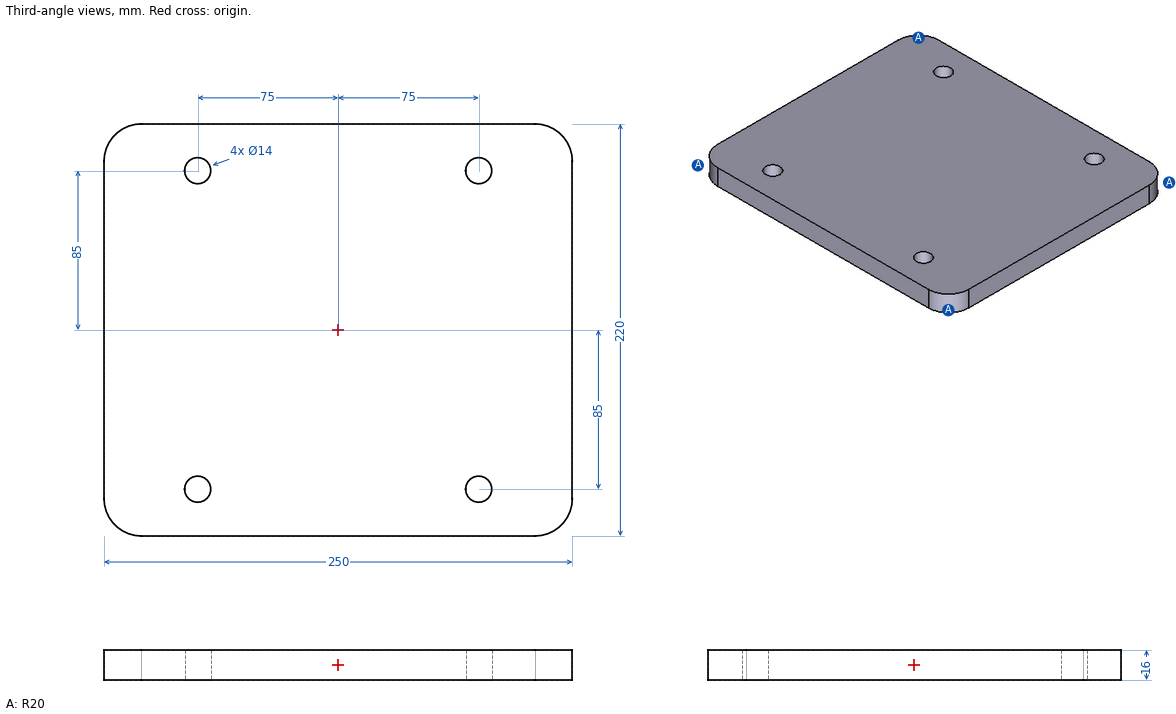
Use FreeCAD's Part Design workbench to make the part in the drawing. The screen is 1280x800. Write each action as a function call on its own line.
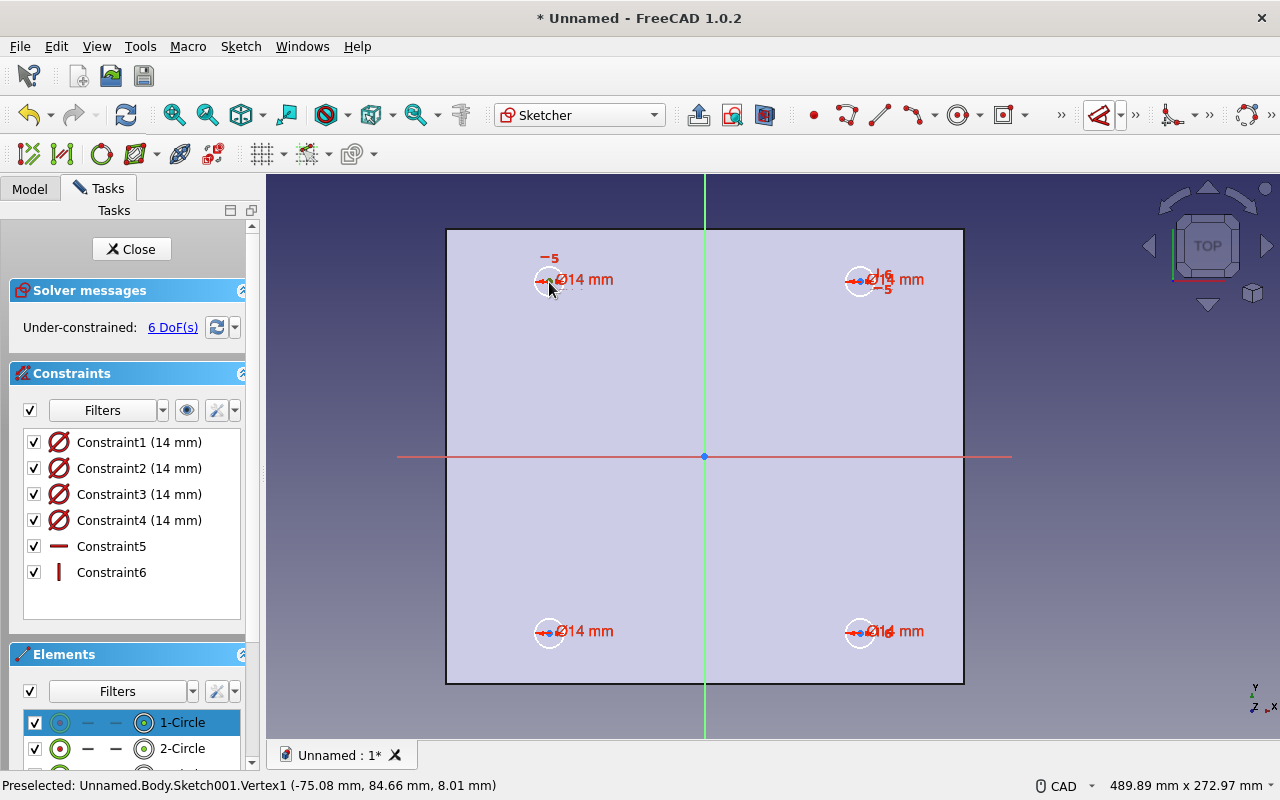
click(550, 633)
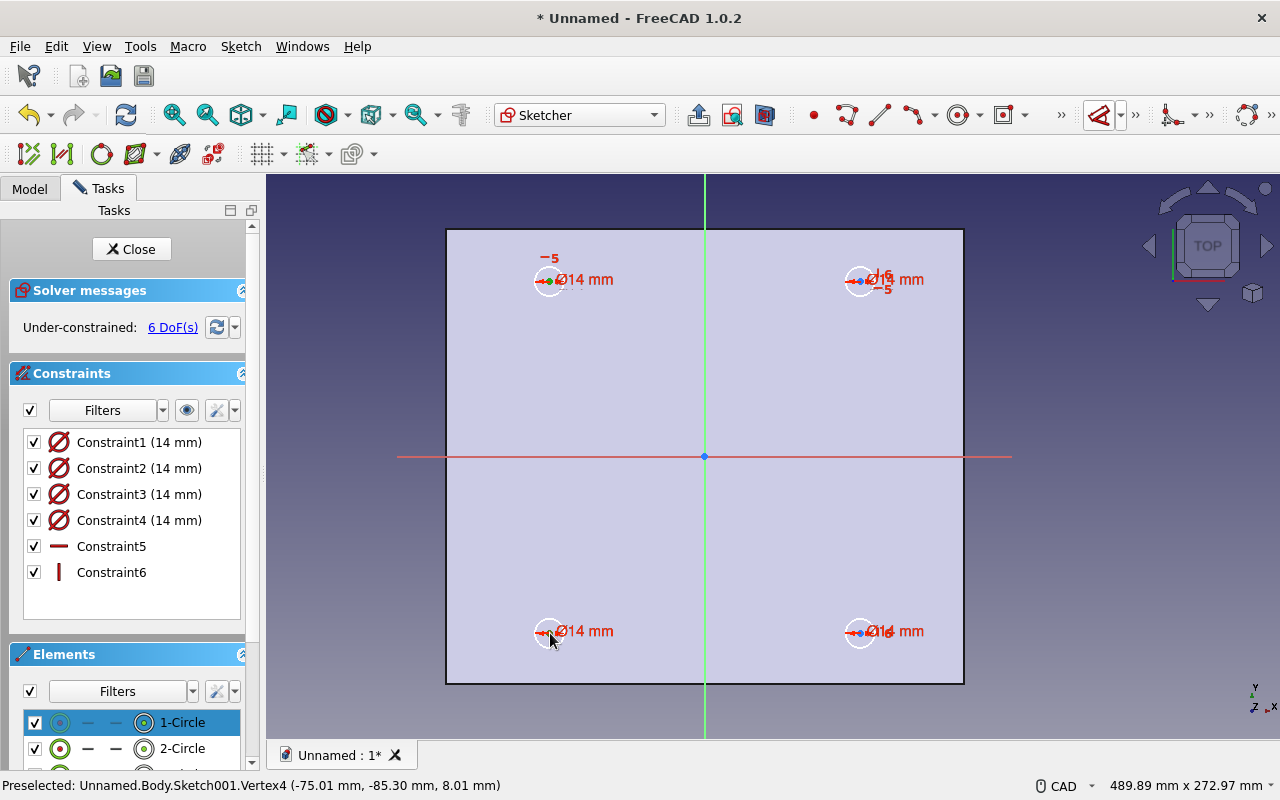
key(v)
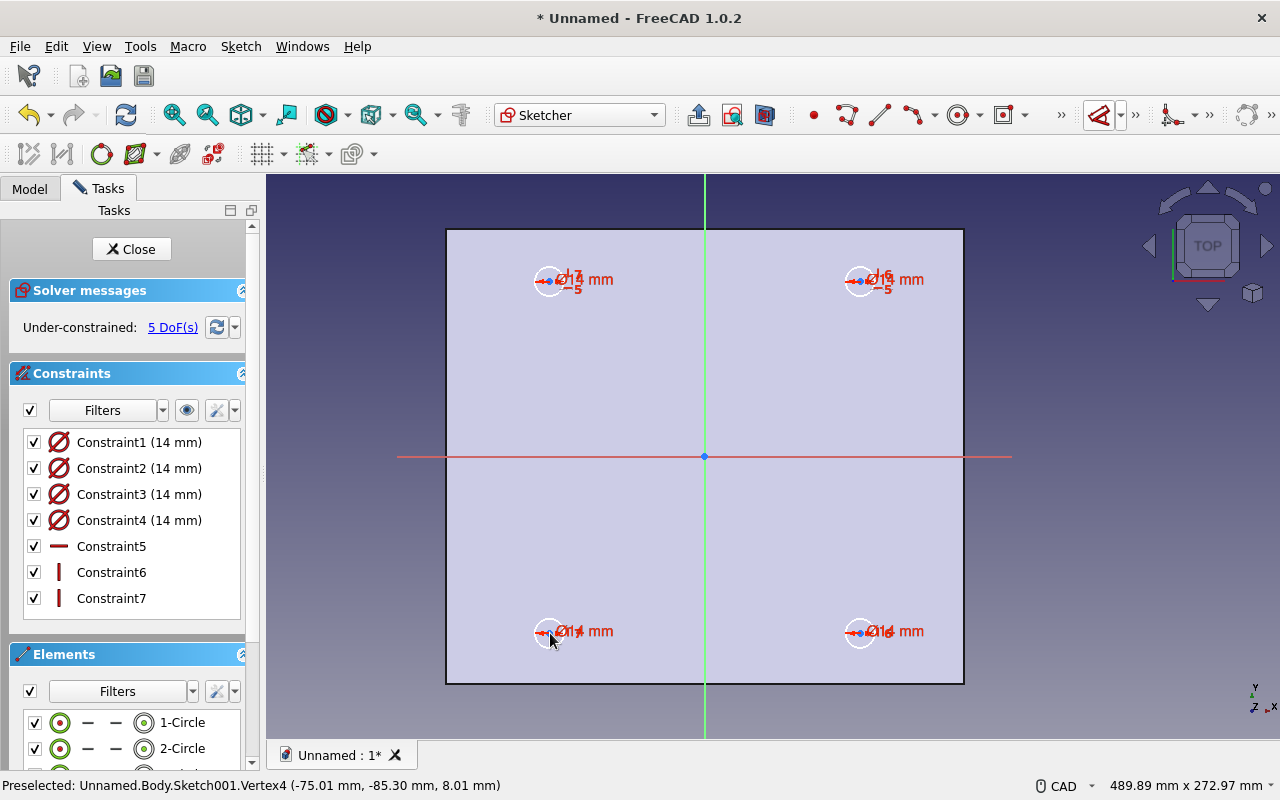
click(860, 633)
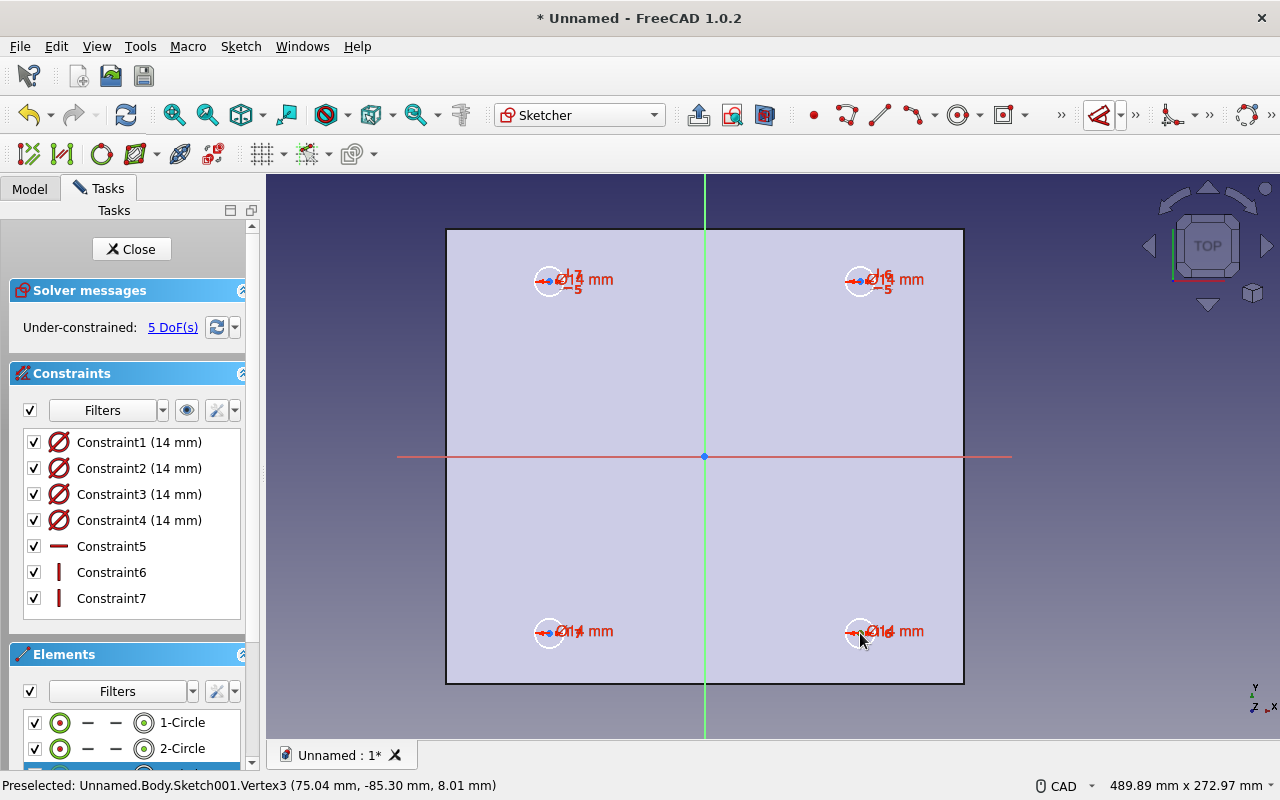
click(549, 633)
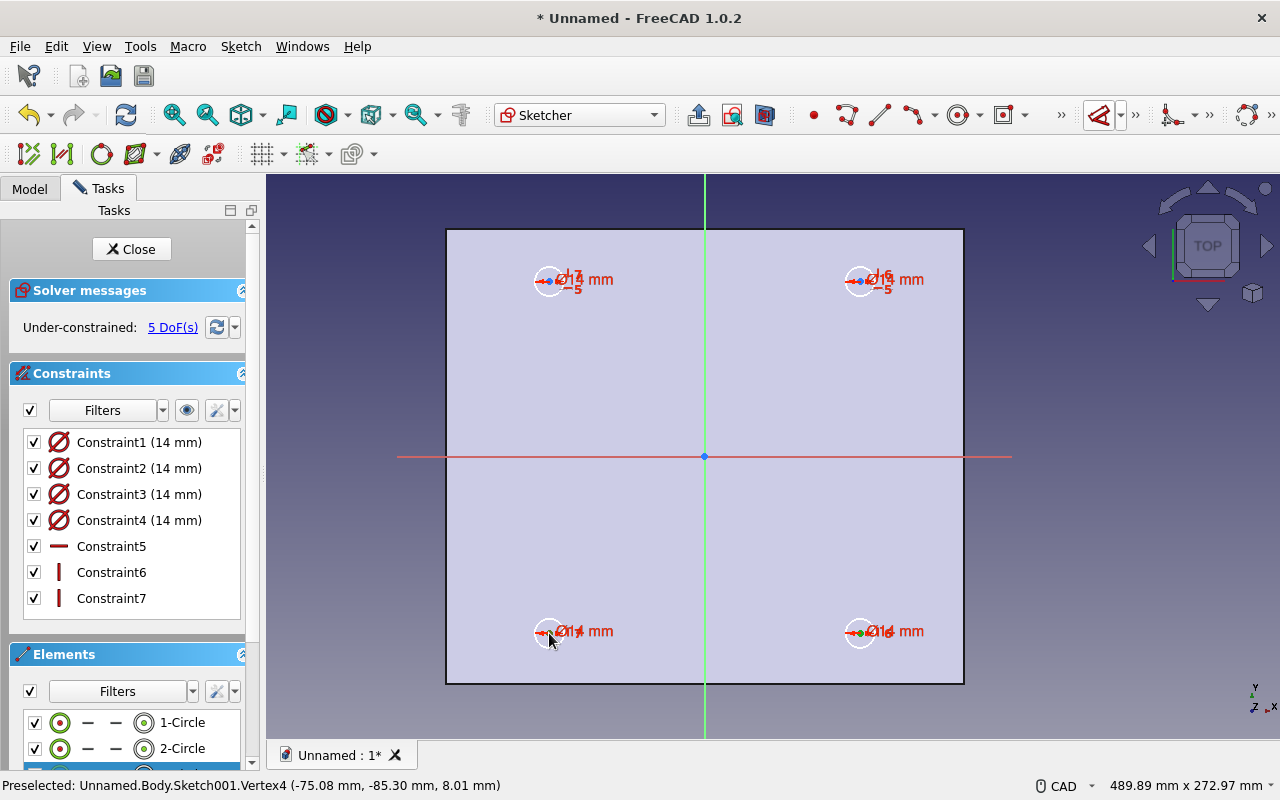
key(h)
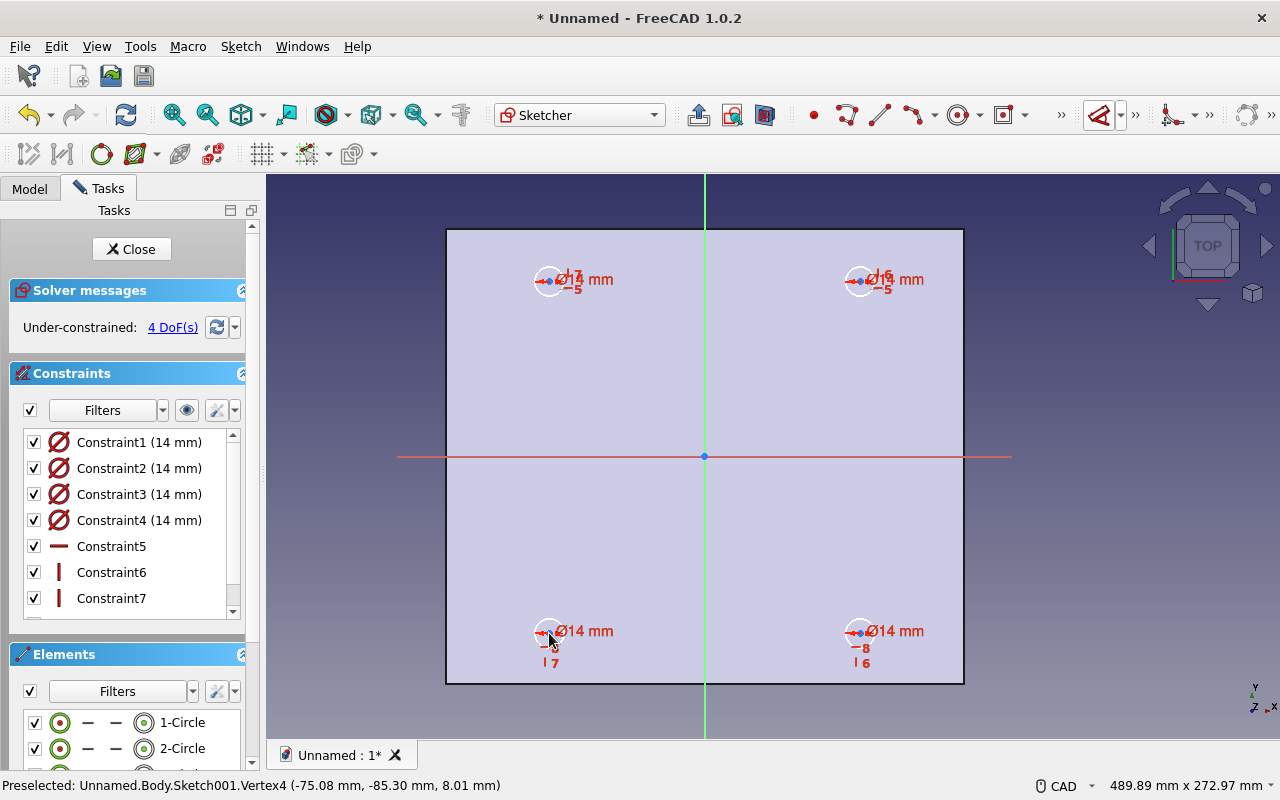
click(549, 282)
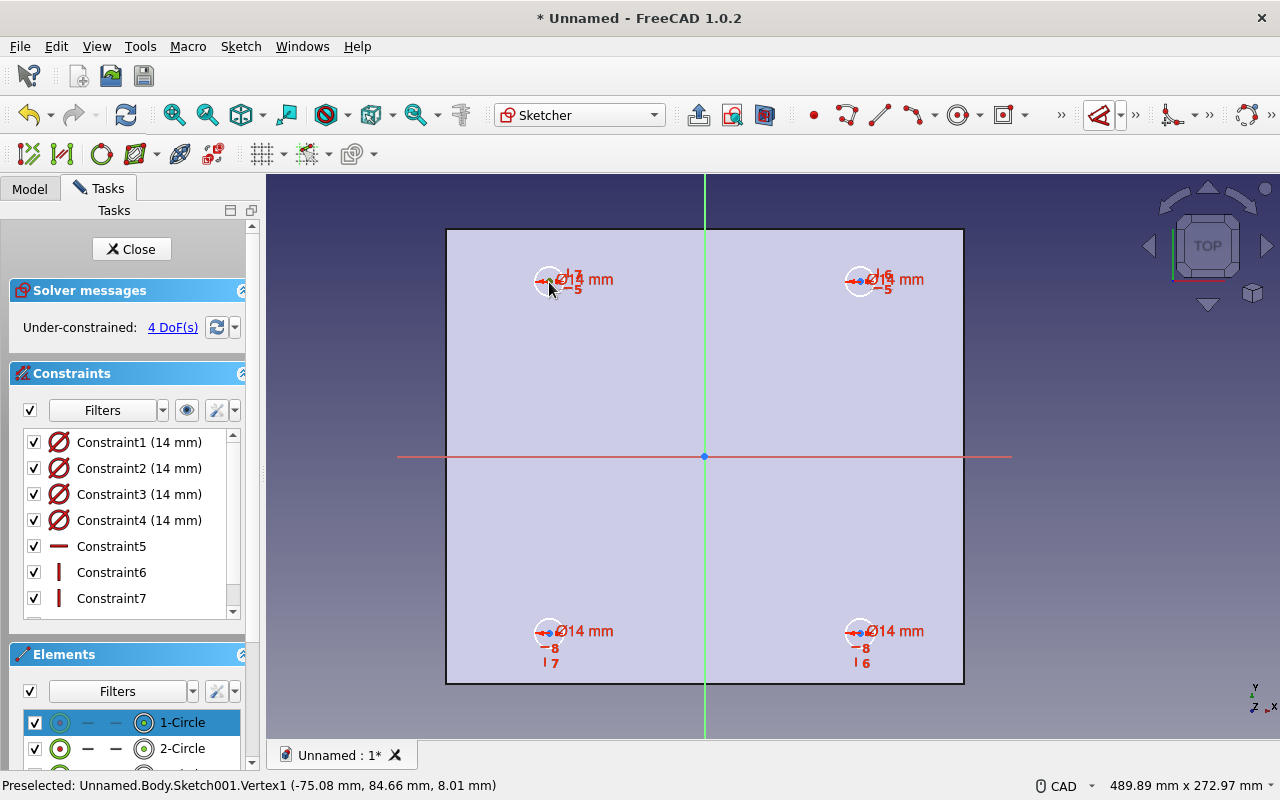
click(1120, 116)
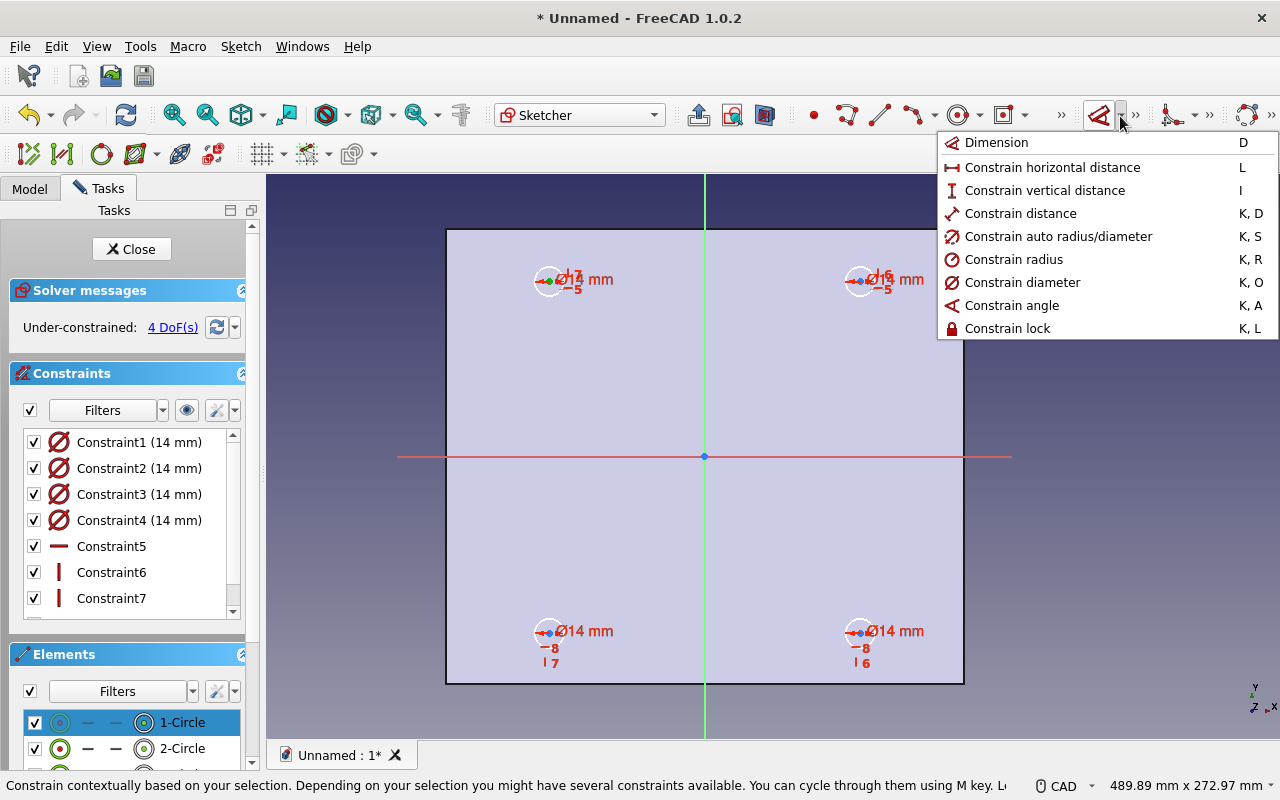
click(1108, 168)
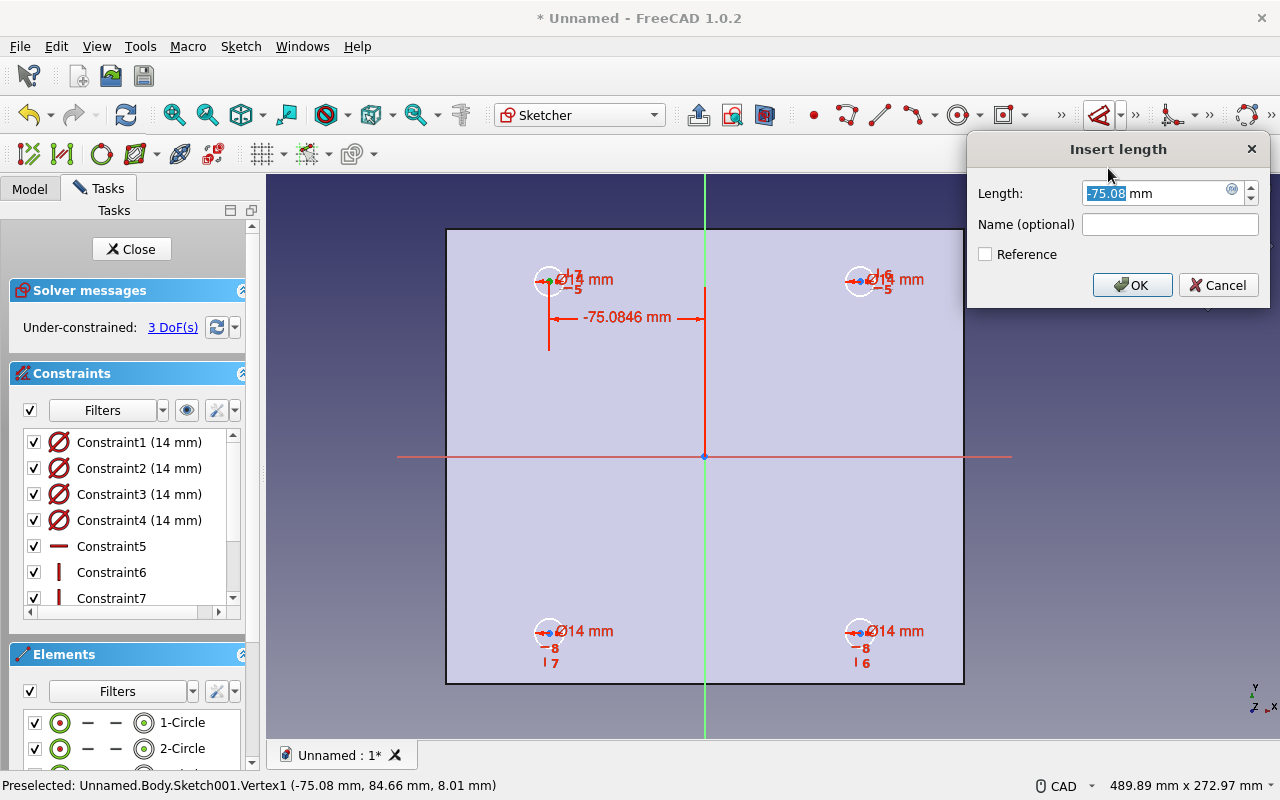
text(-75)
key(Return)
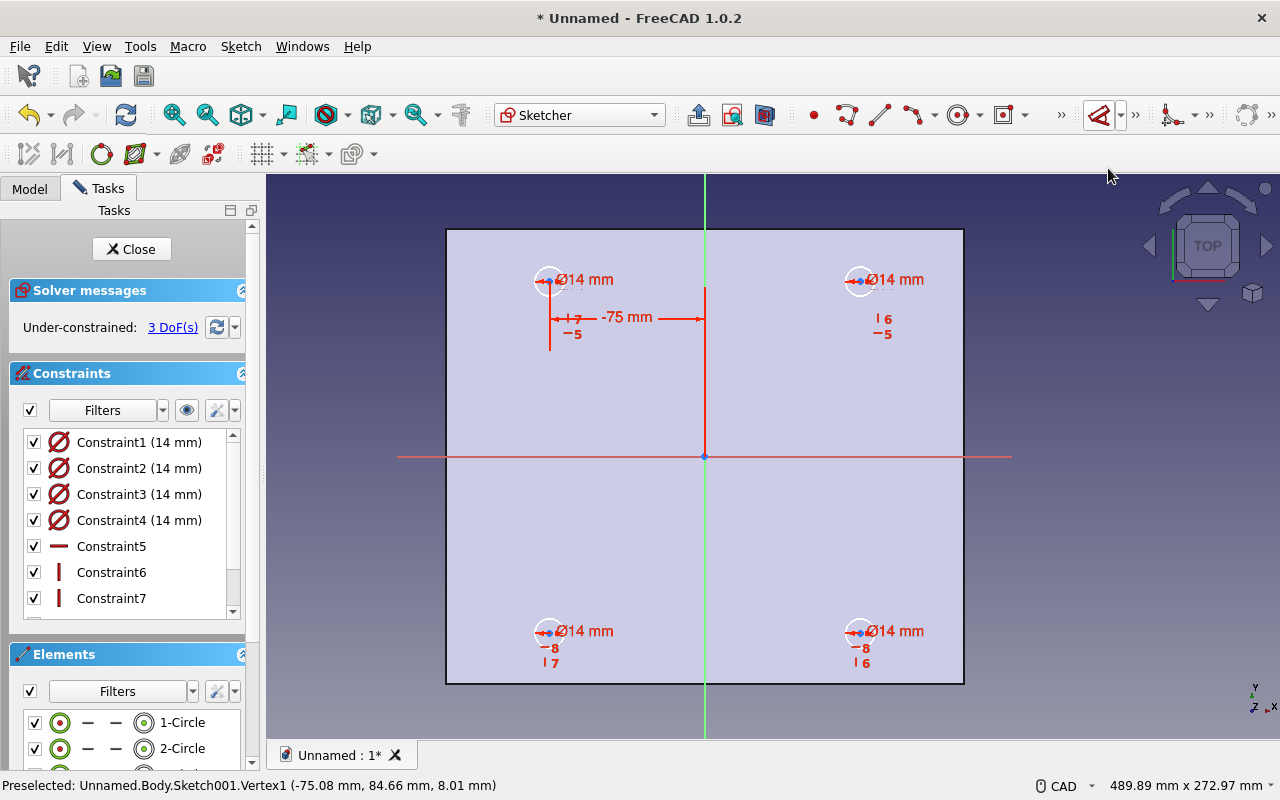
click(550, 282)